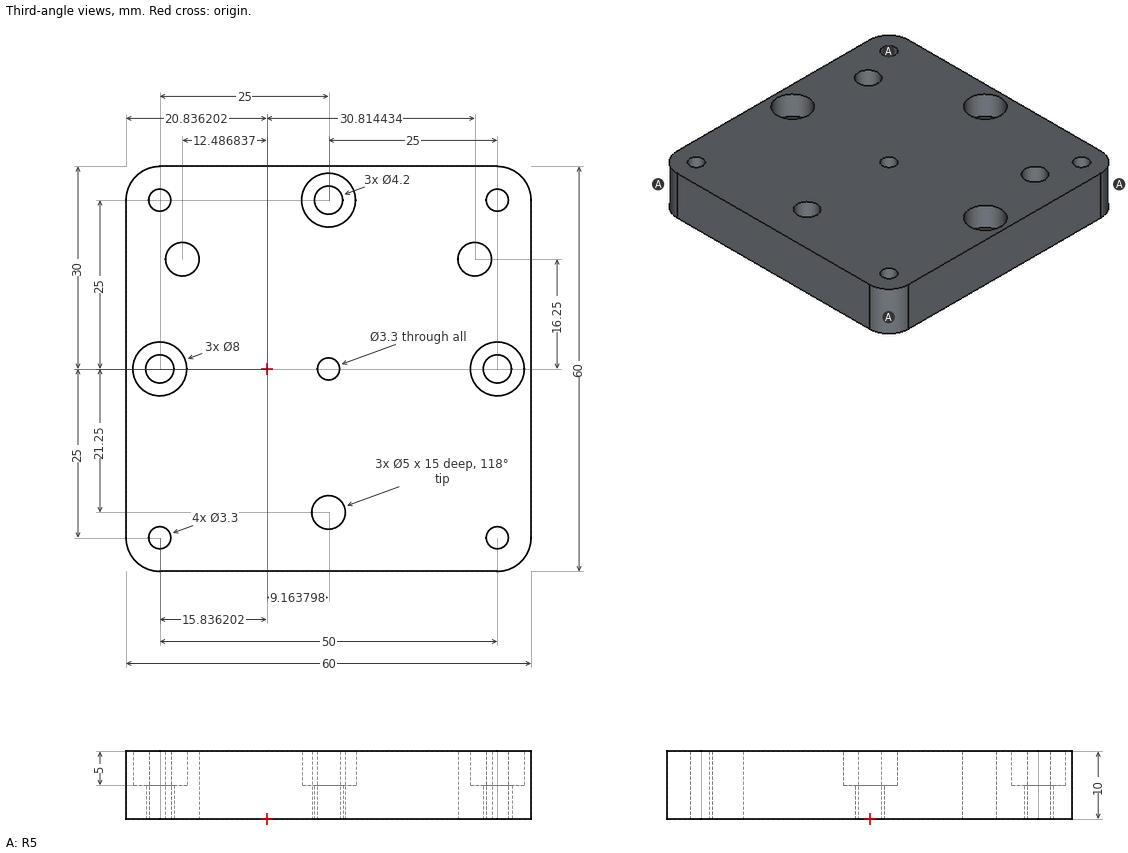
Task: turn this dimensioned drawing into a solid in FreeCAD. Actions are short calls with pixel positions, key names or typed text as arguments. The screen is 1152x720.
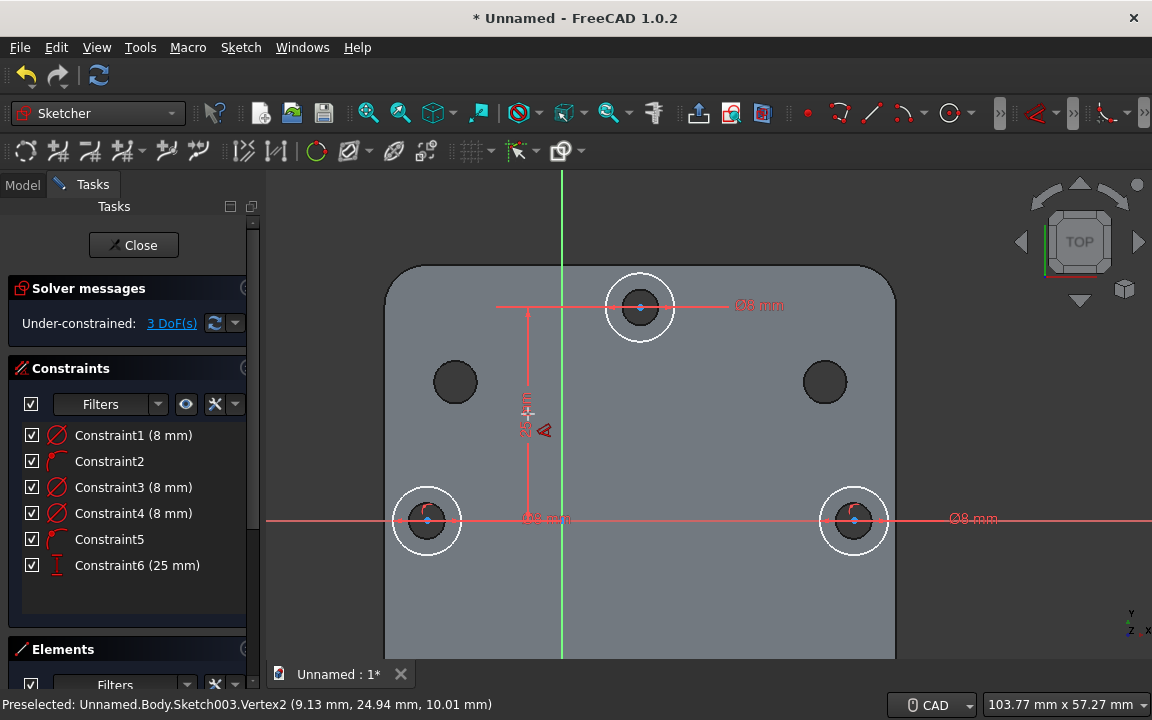
click(427, 521)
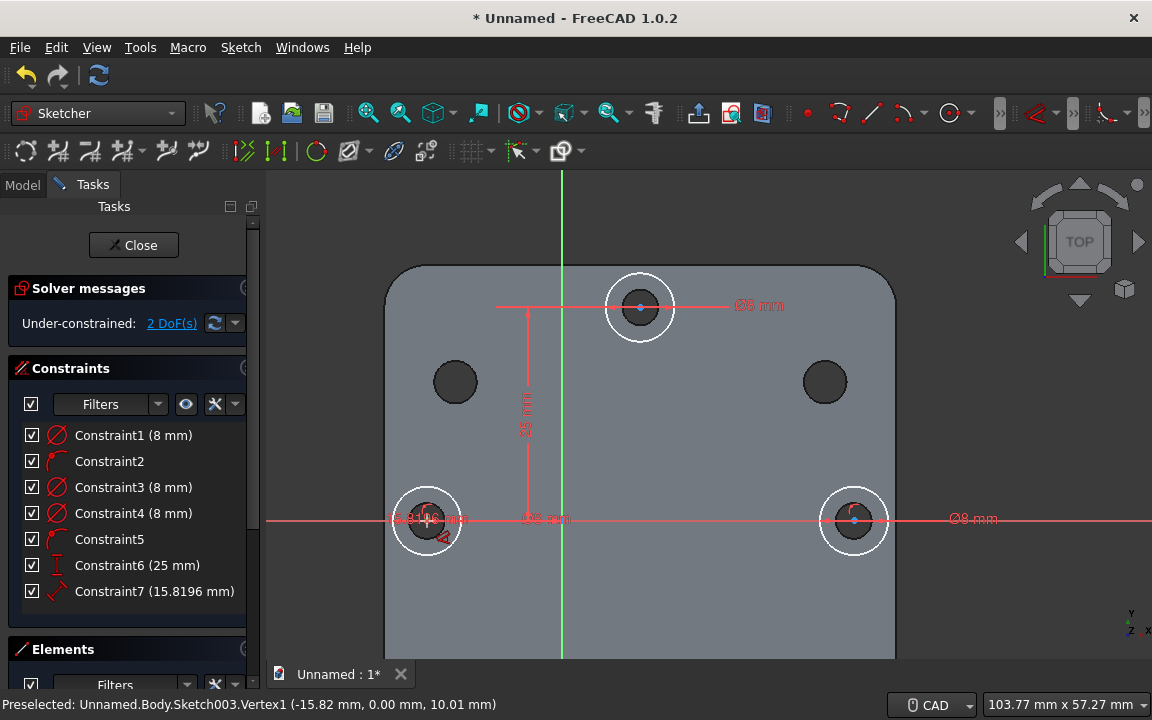
click(640, 307)
click(534, 555)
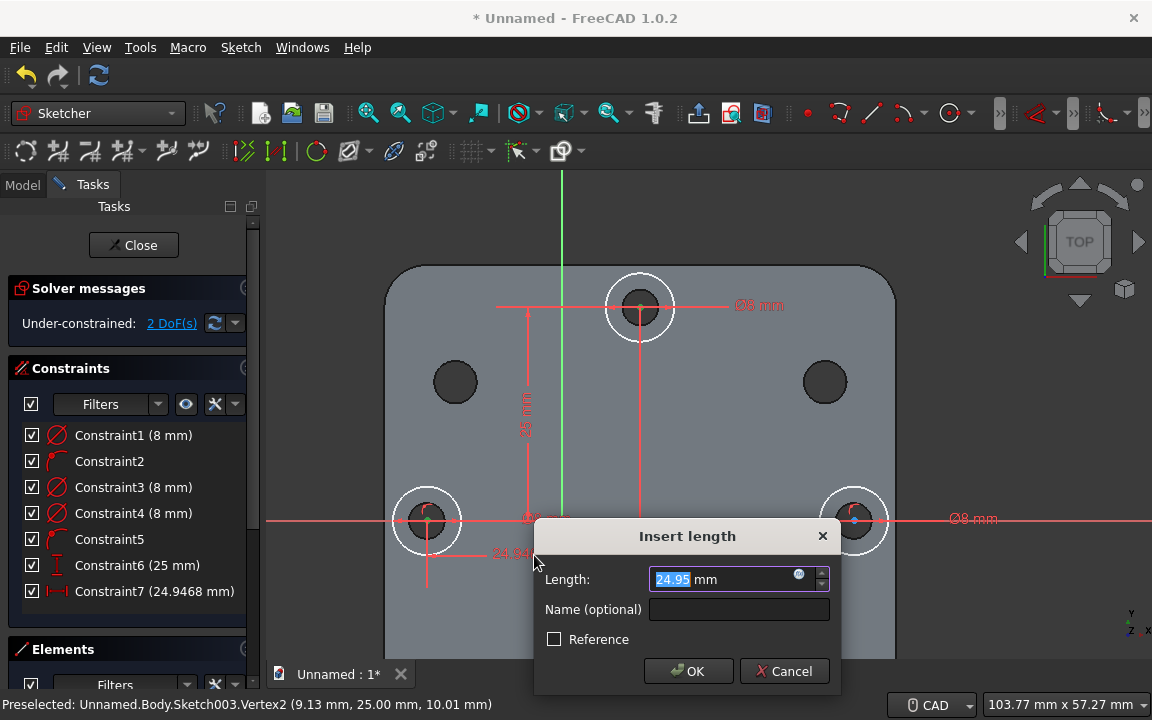
text(25)
key(Return)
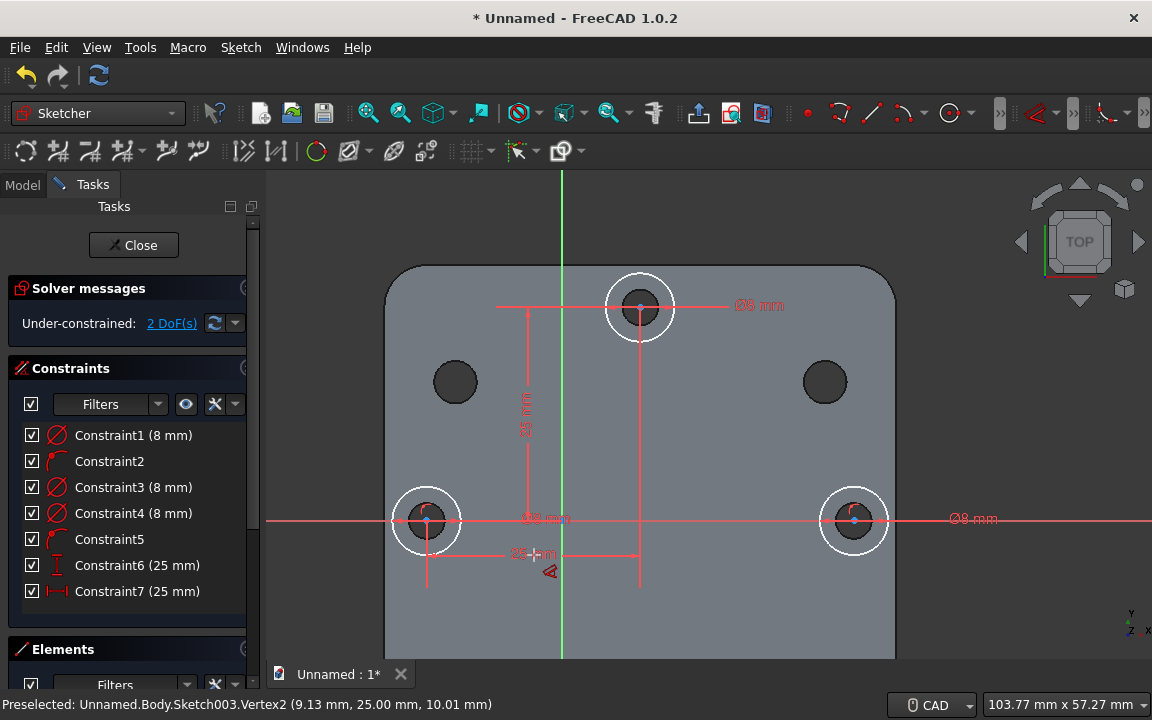
click(640, 307)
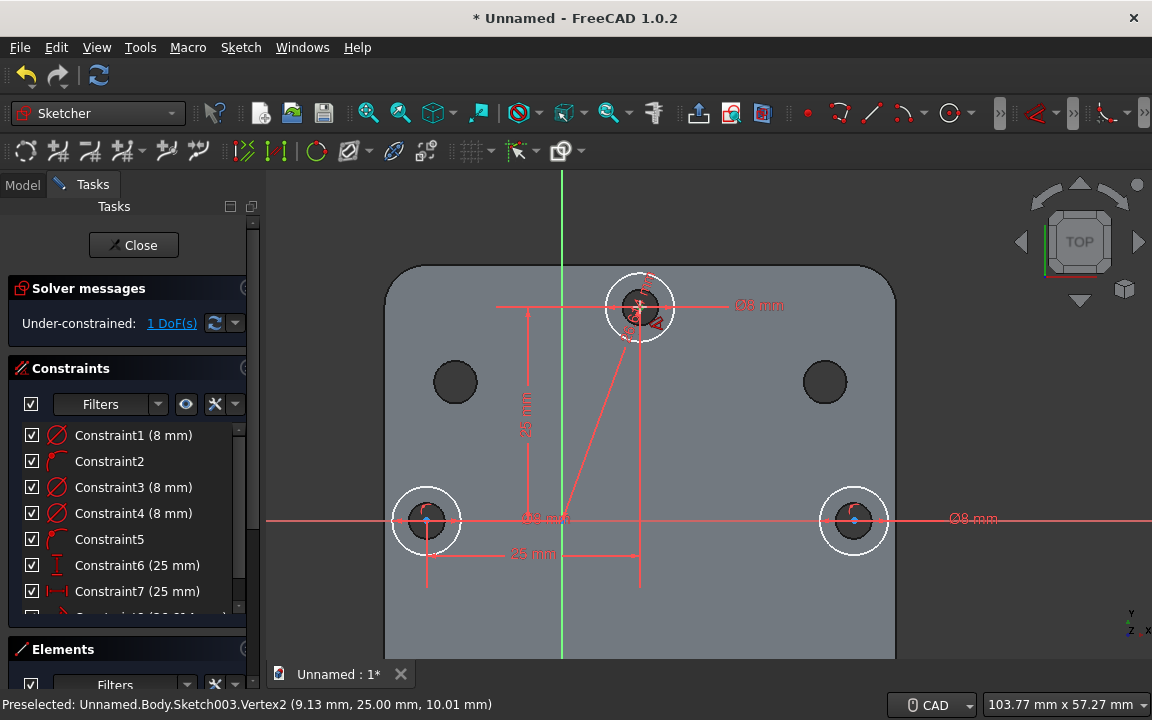
click(854, 521)
click(747, 555)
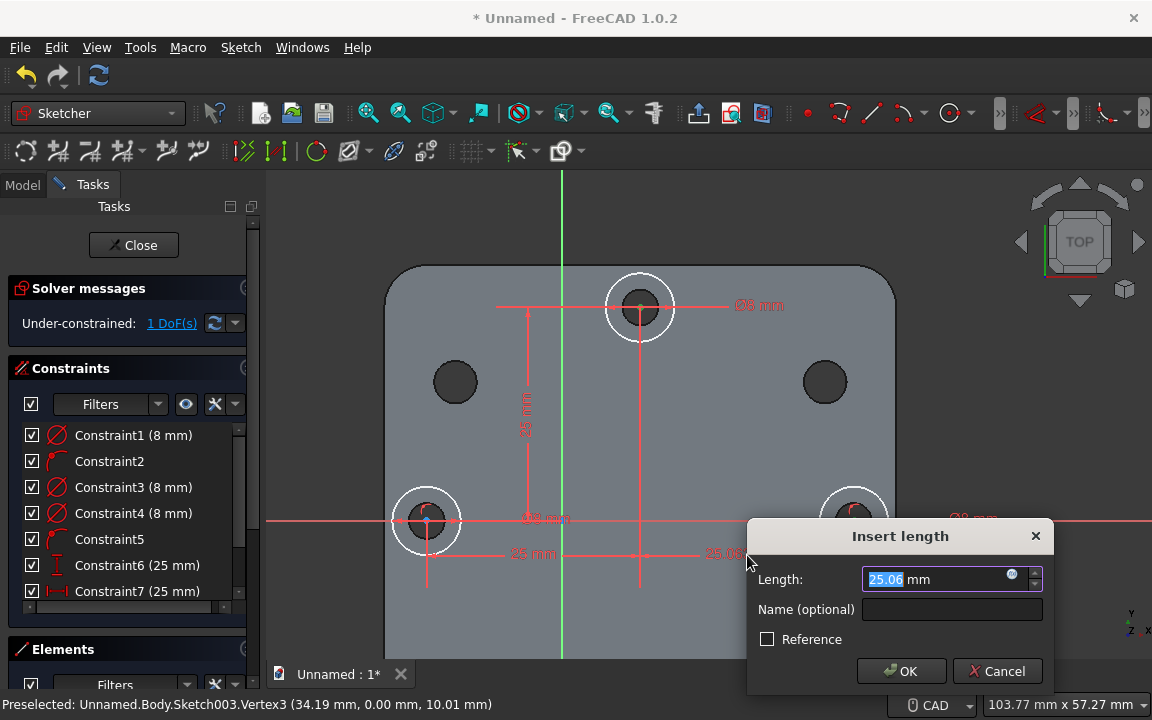
text(25)
key(Return)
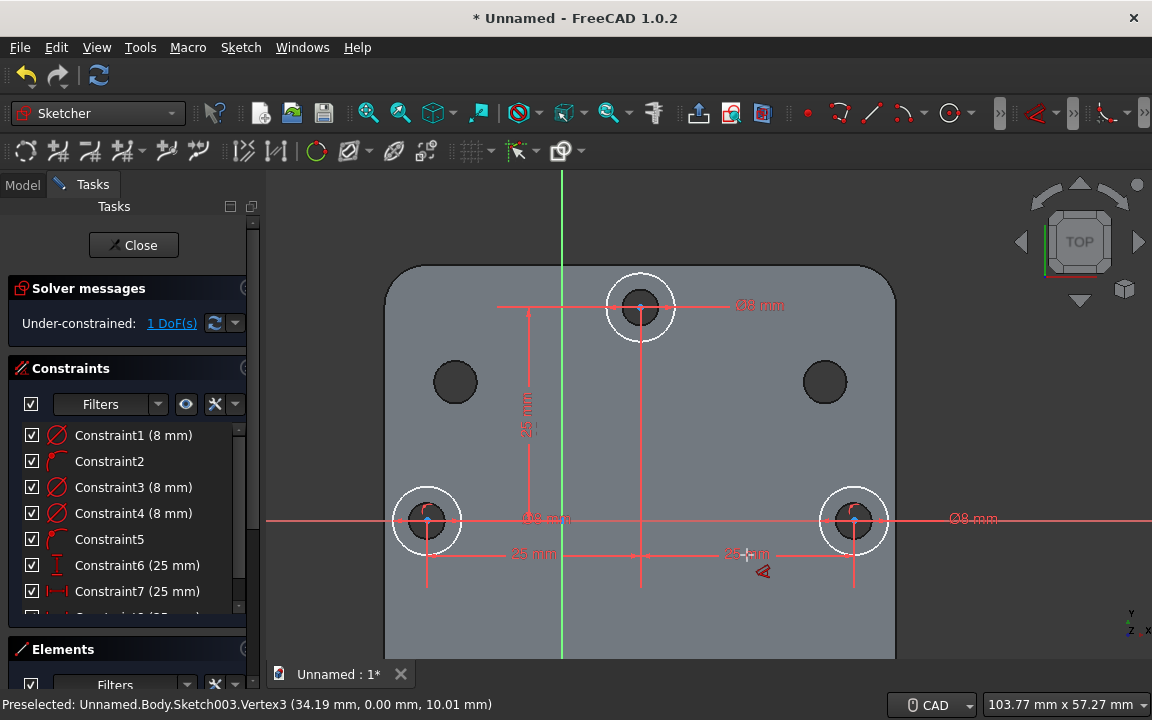
click(641, 307)
click(619, 555)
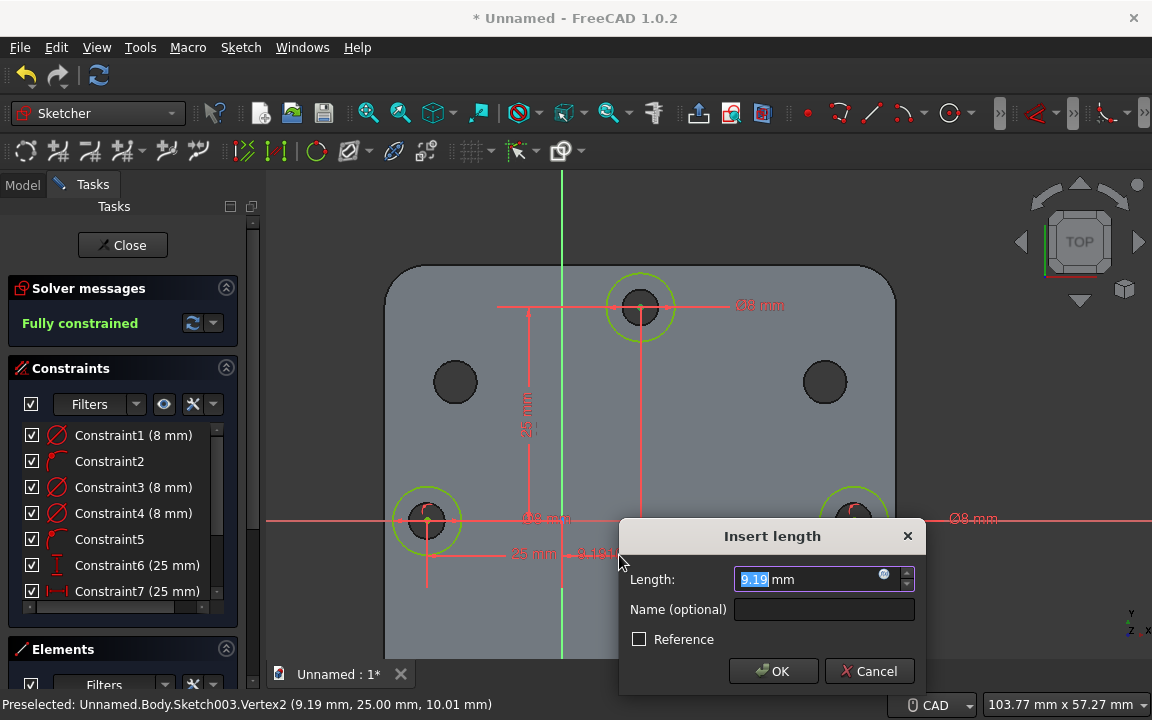
text(9.163798)
key(Return)
key(Escape)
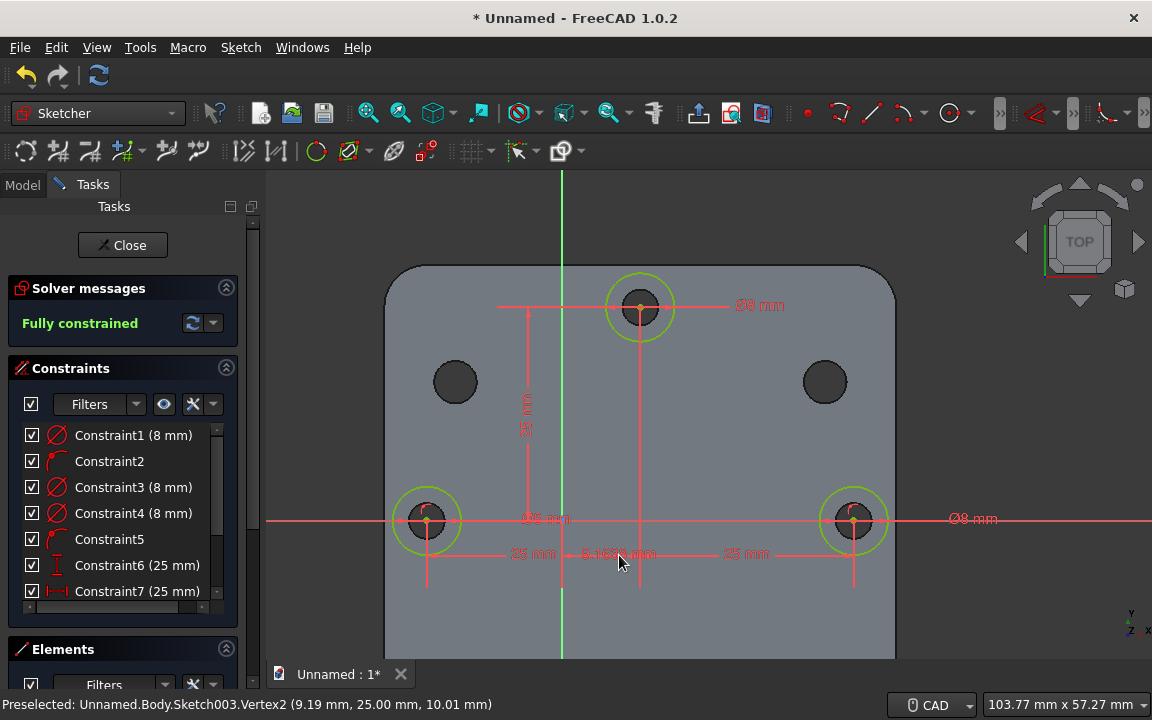
click(123, 245)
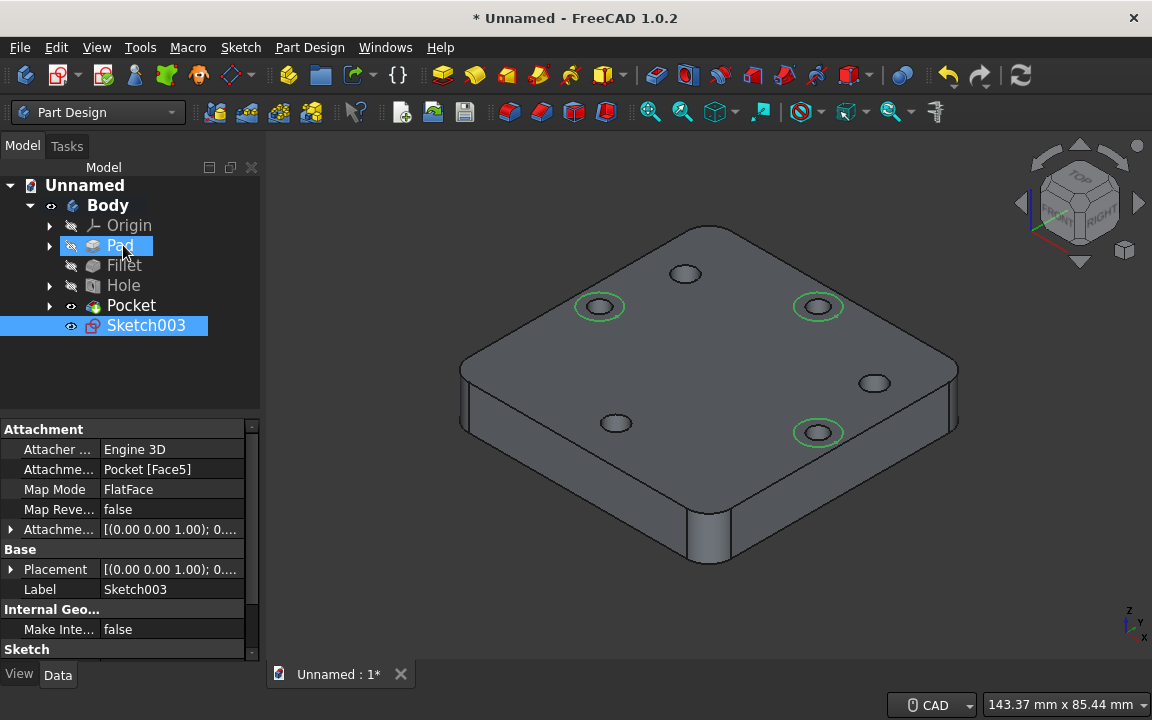
click(658, 76)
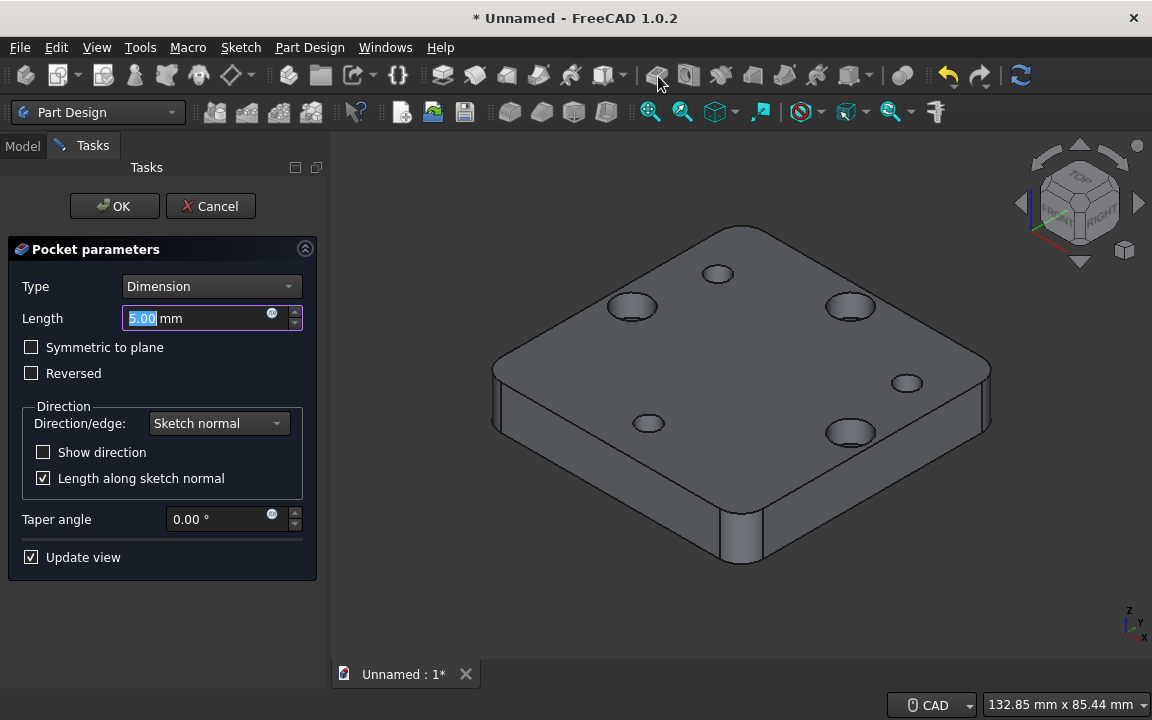
text(5)
key(Tab)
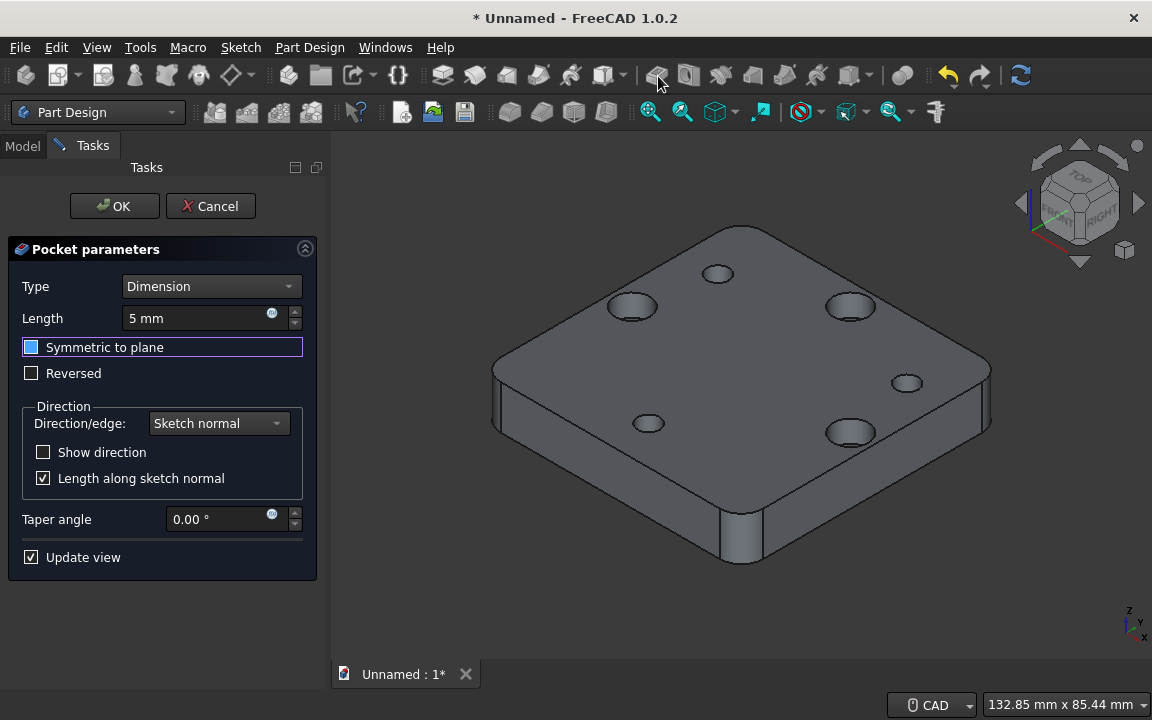
click(115, 206)